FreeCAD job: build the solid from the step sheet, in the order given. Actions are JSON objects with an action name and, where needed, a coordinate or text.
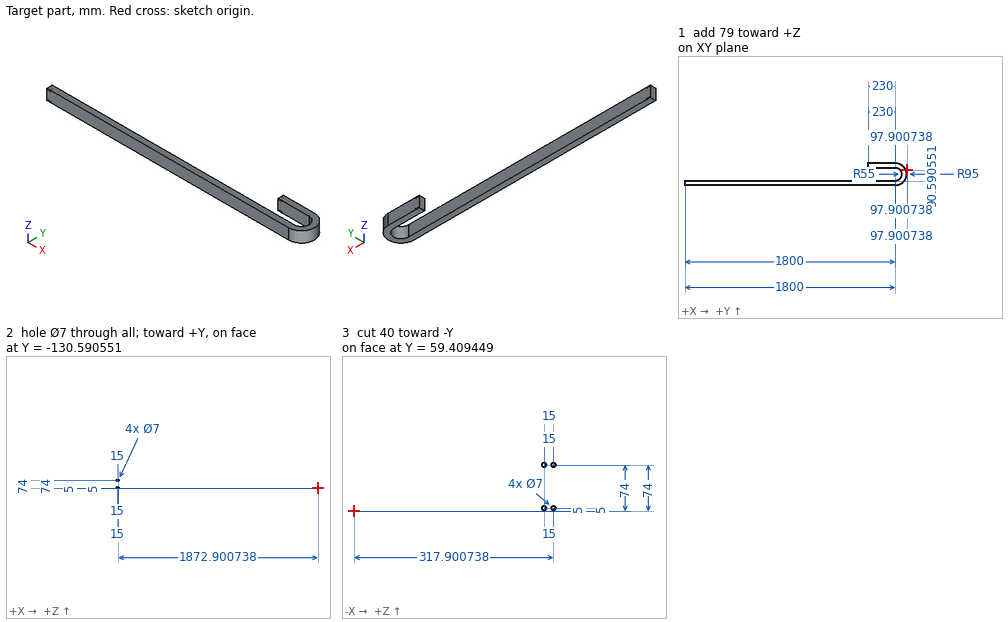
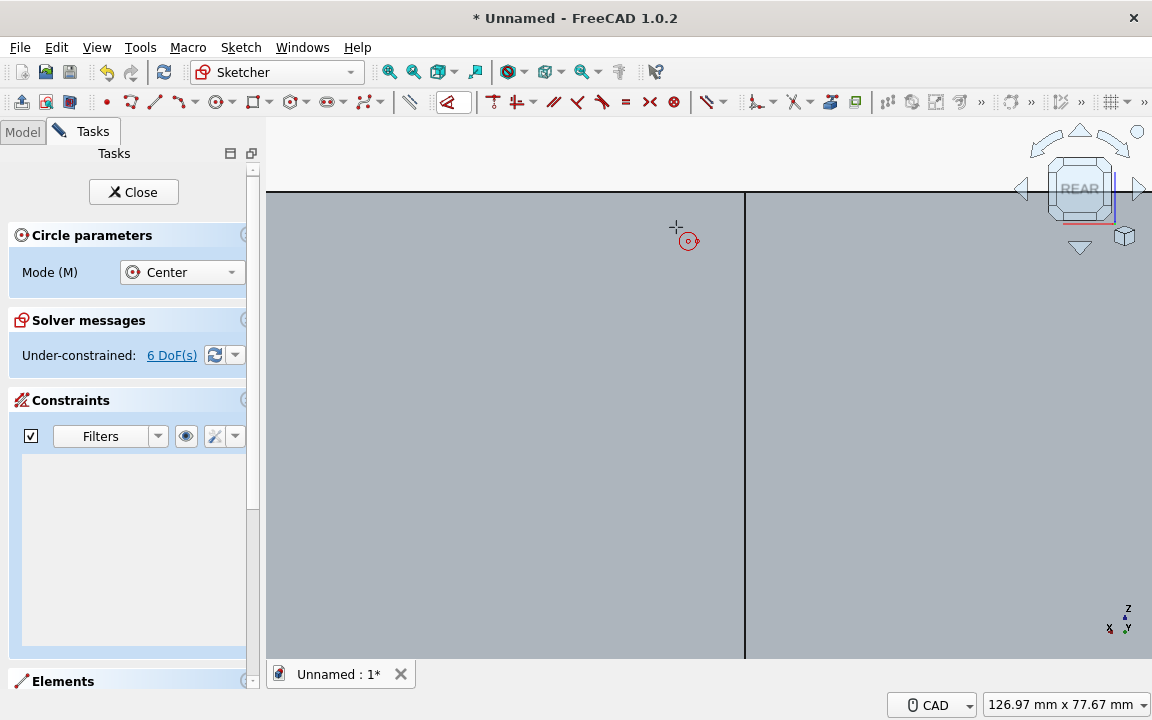
{"action": "left_click", "coordinate": [676, 227]}
{"action": "left_click", "coordinate": [693, 209]}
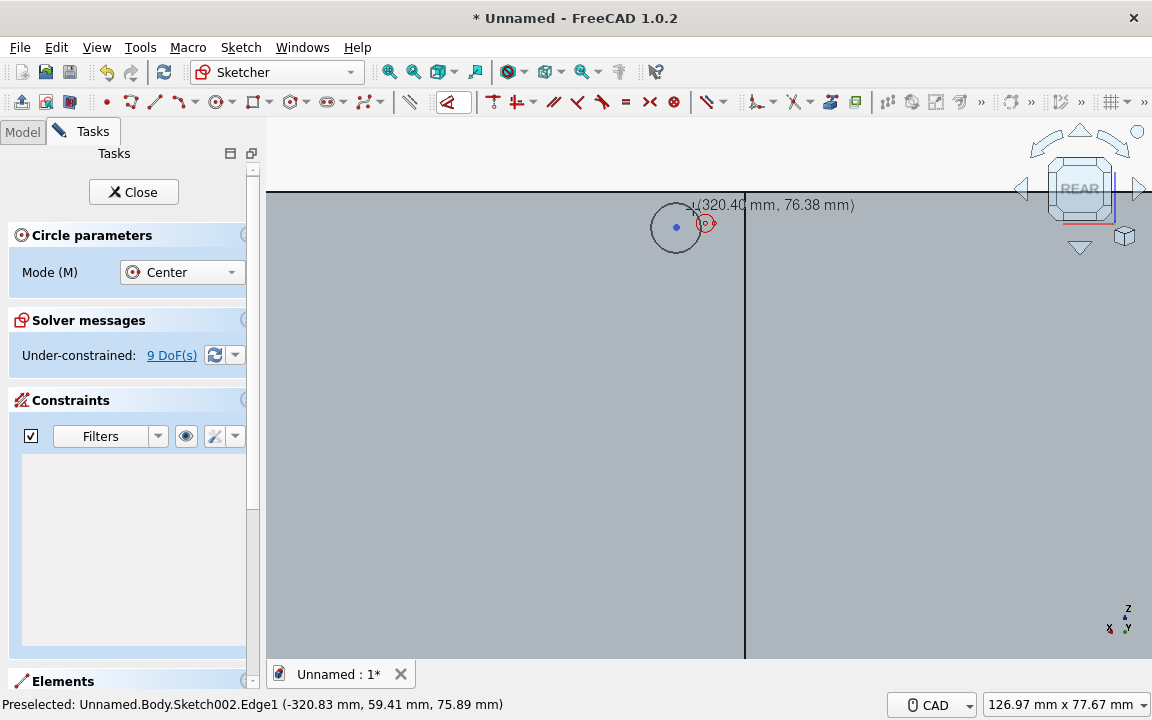
{"action": "left_click", "coordinate": [571, 227]}
{"action": "left_click", "coordinate": [588, 209]}
{"action": "key", "text": "Escape"}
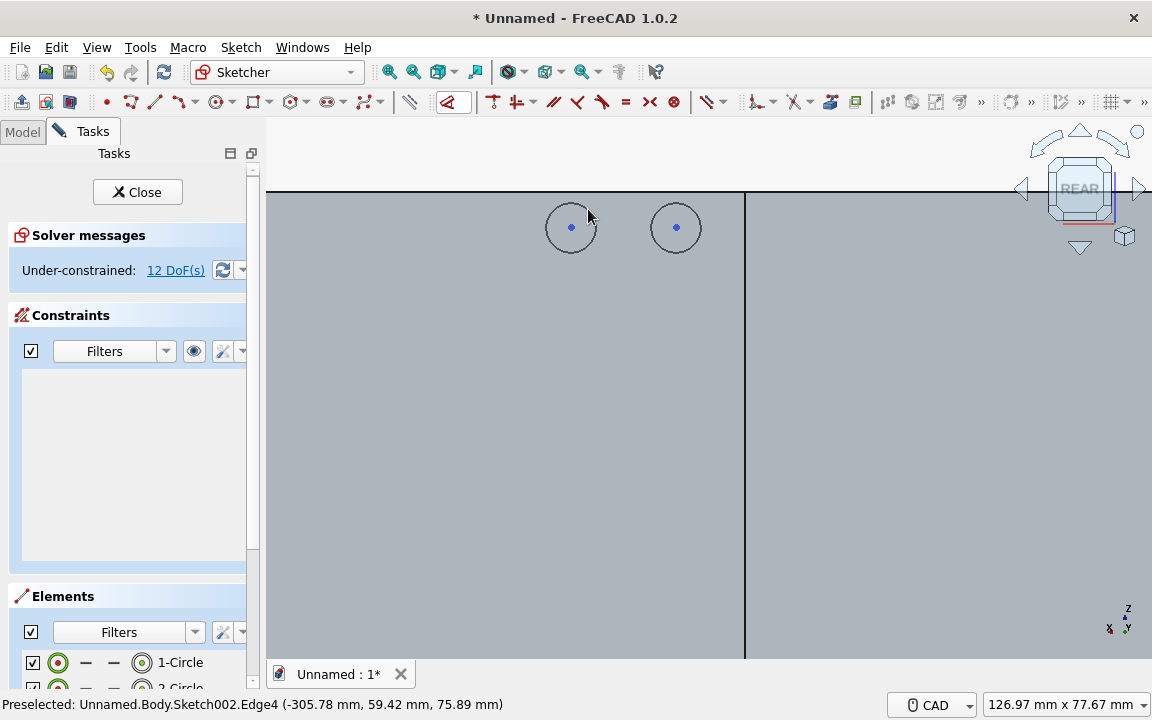
{"action": "scroll", "coordinate": [676, 227], "scroll_direction": "down", "scroll_amount": 2}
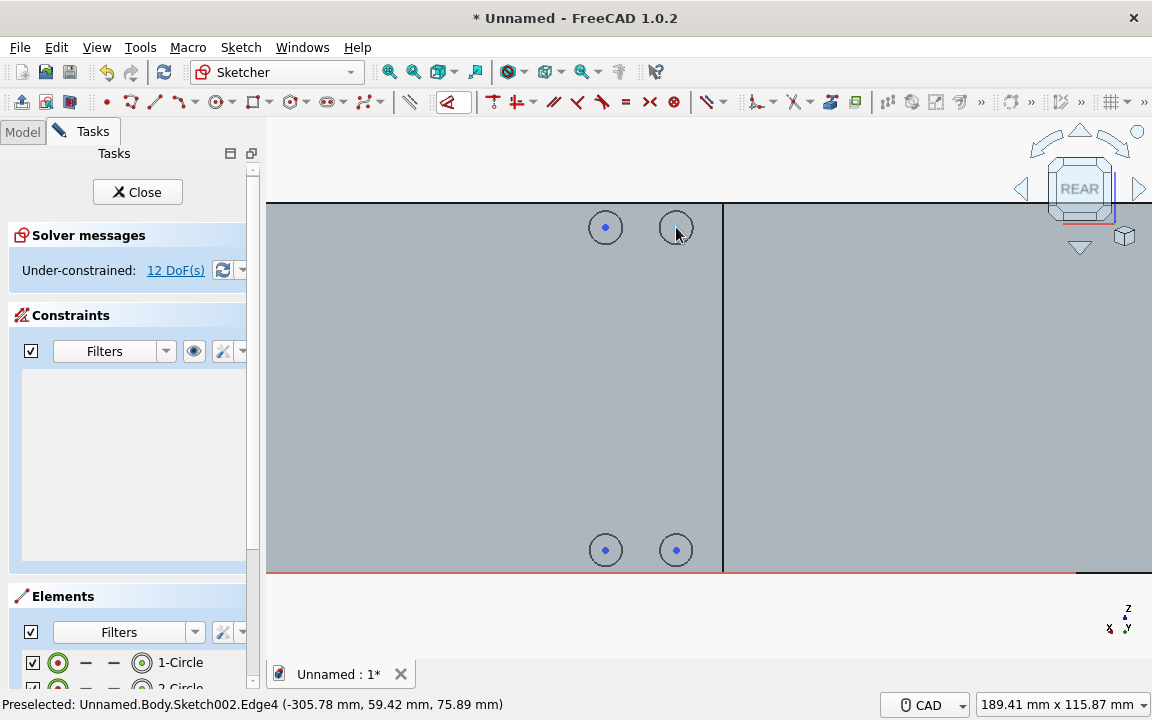
{"action": "left_click", "coordinate": [688, 539]}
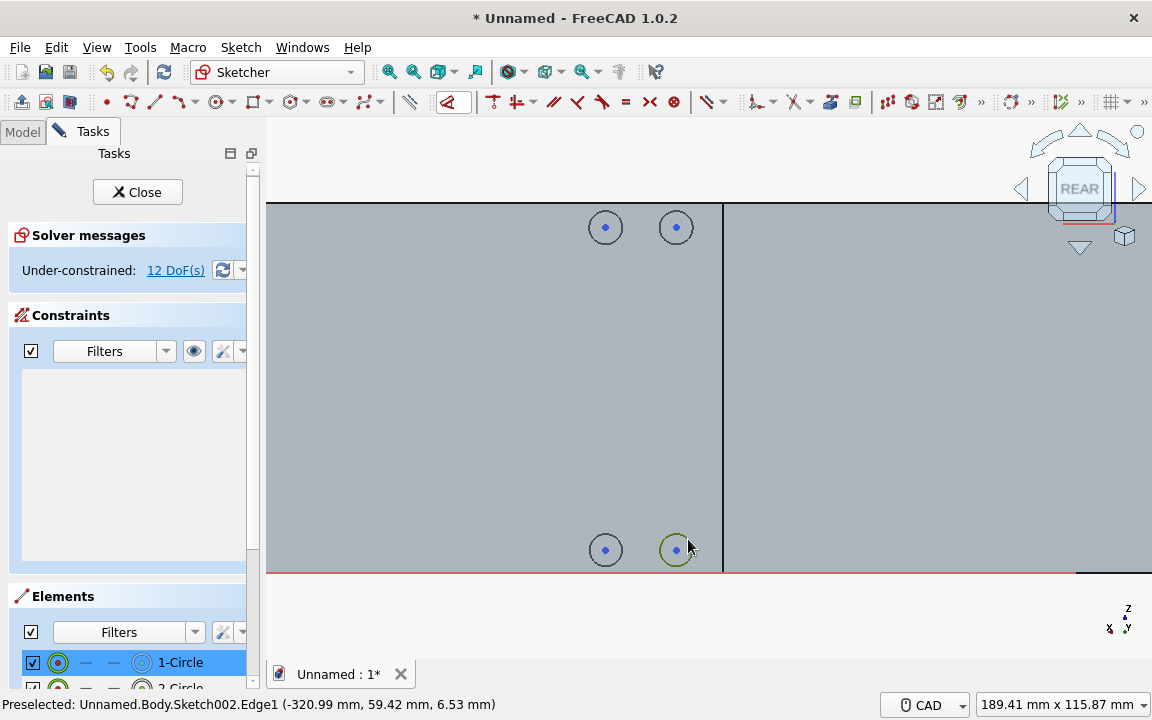
{"action": "left_click", "coordinate": [617, 539]}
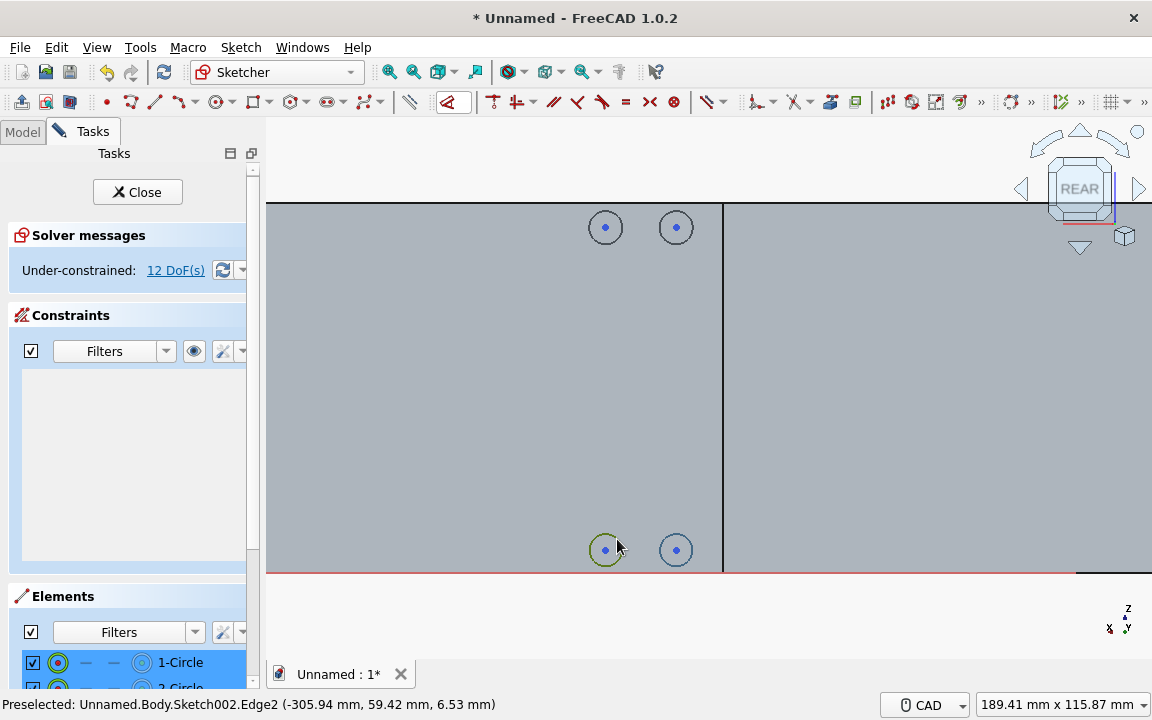
{"action": "left_click", "coordinate": [688, 216]}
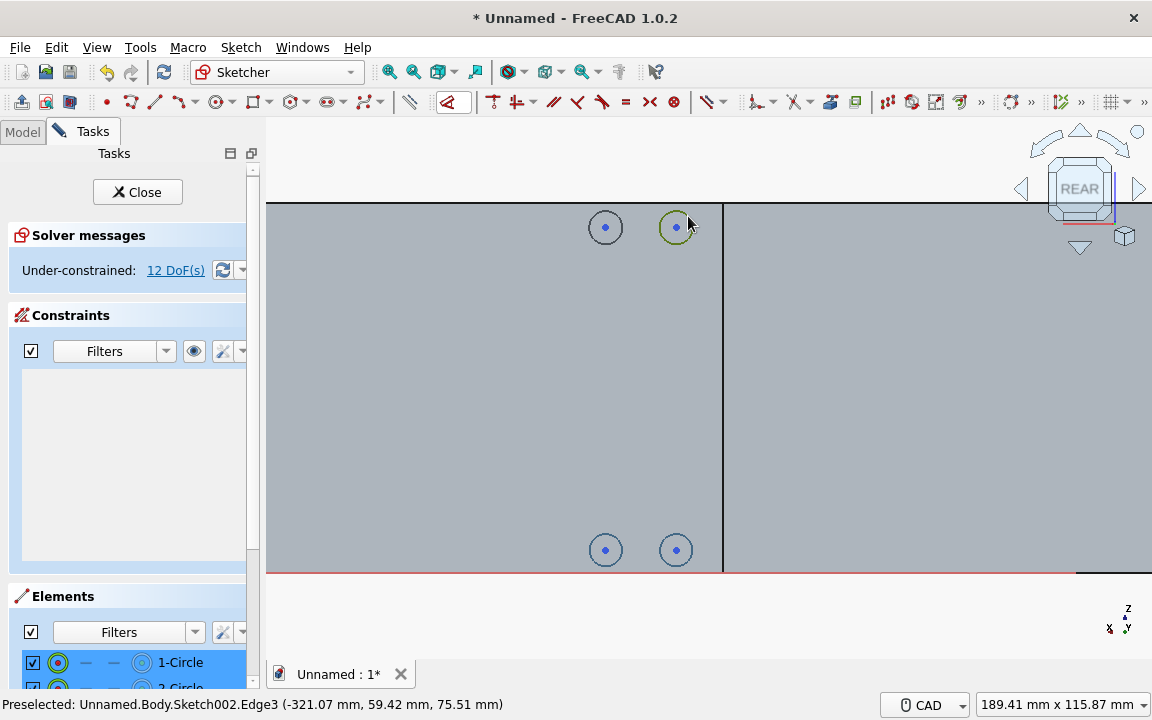
{"action": "left_click", "coordinate": [617, 216]}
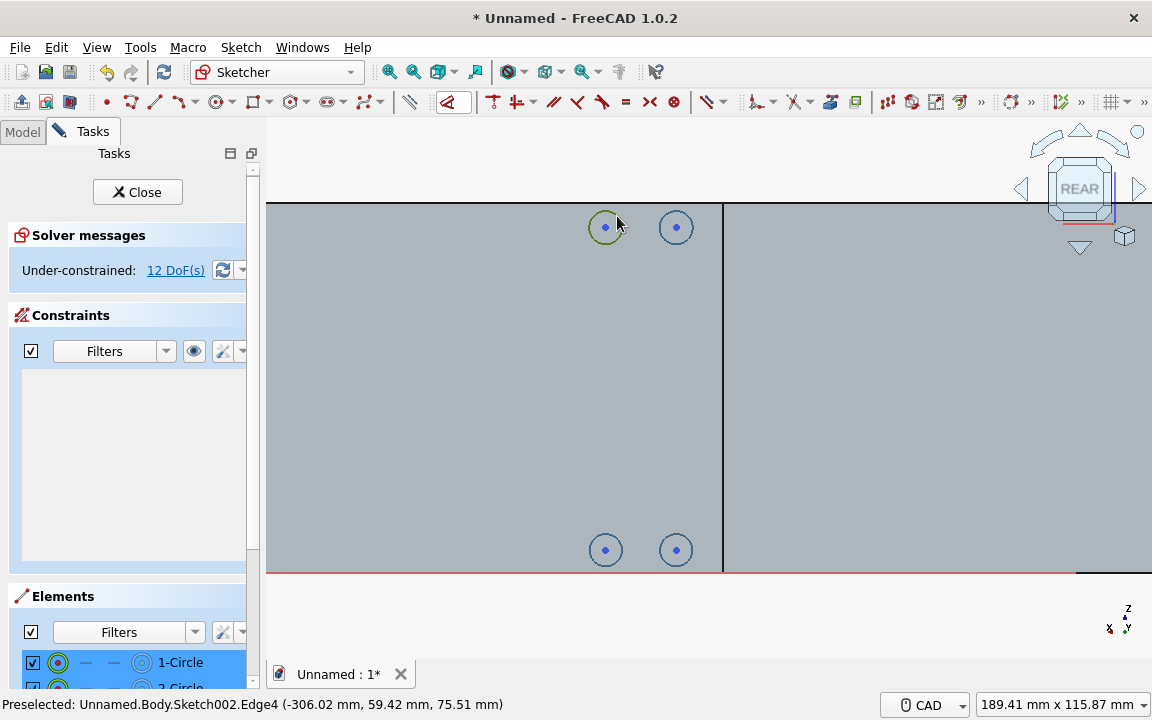
{"action": "key", "text": "e"}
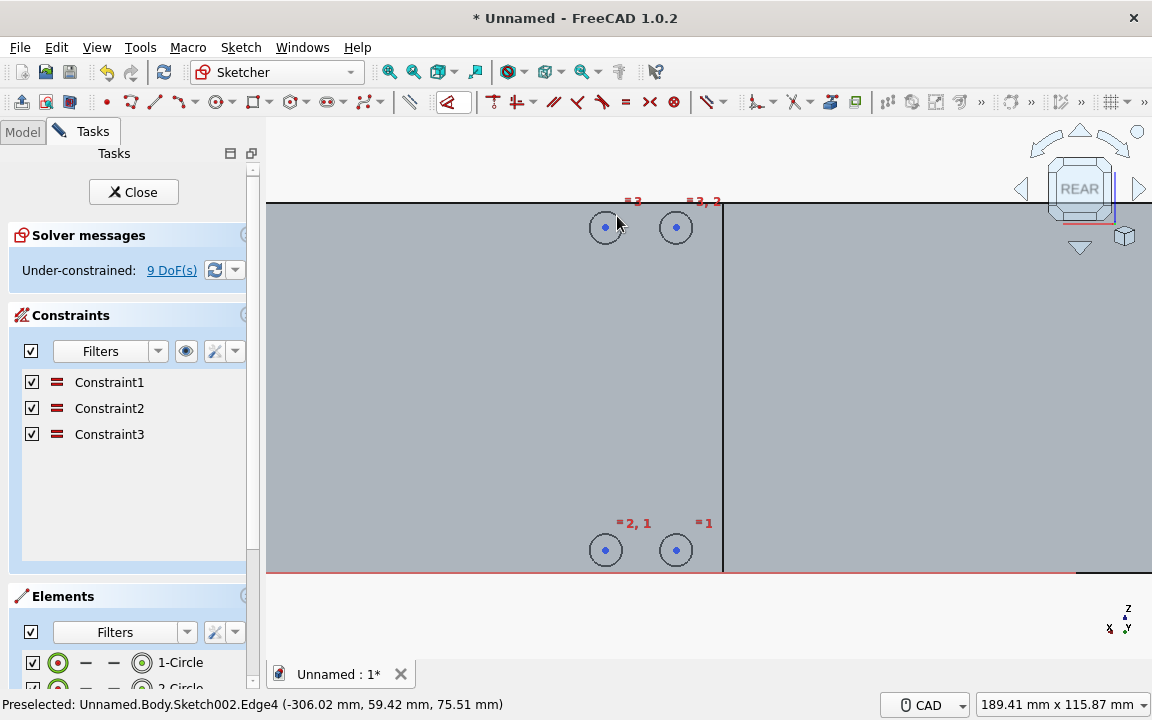
{"action": "key", "text": "d"}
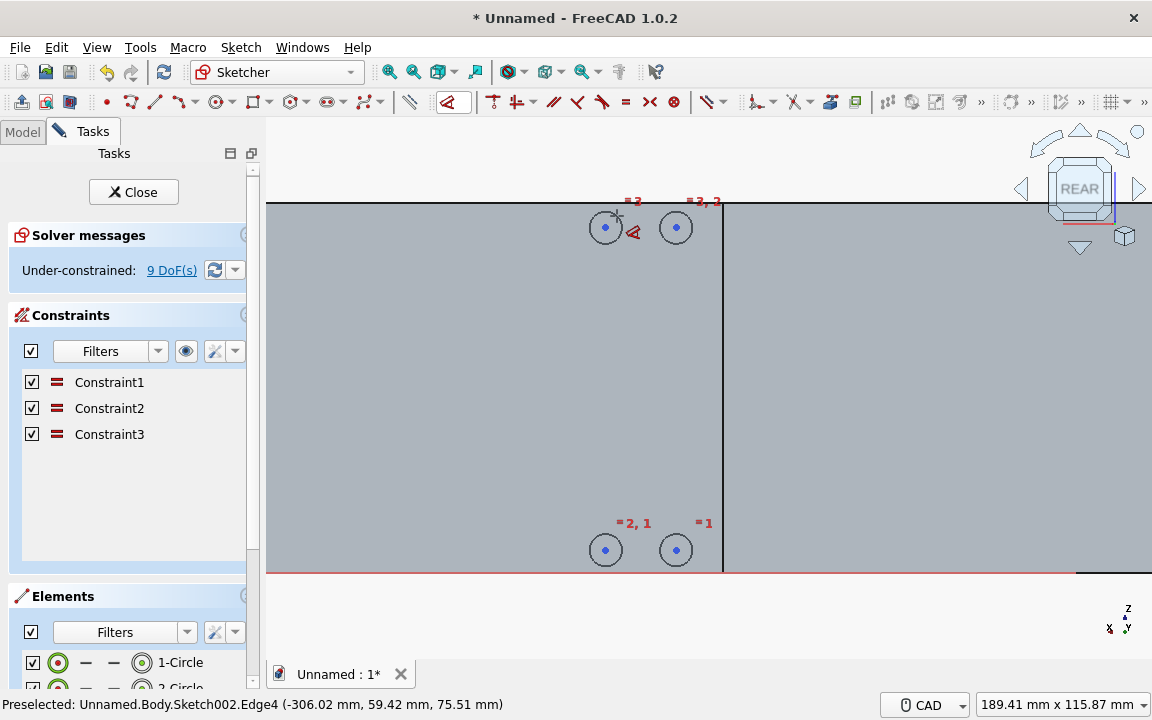
{"action": "left_click", "coordinate": [688, 539]}
{"action": "left_click", "coordinate": [711, 517]}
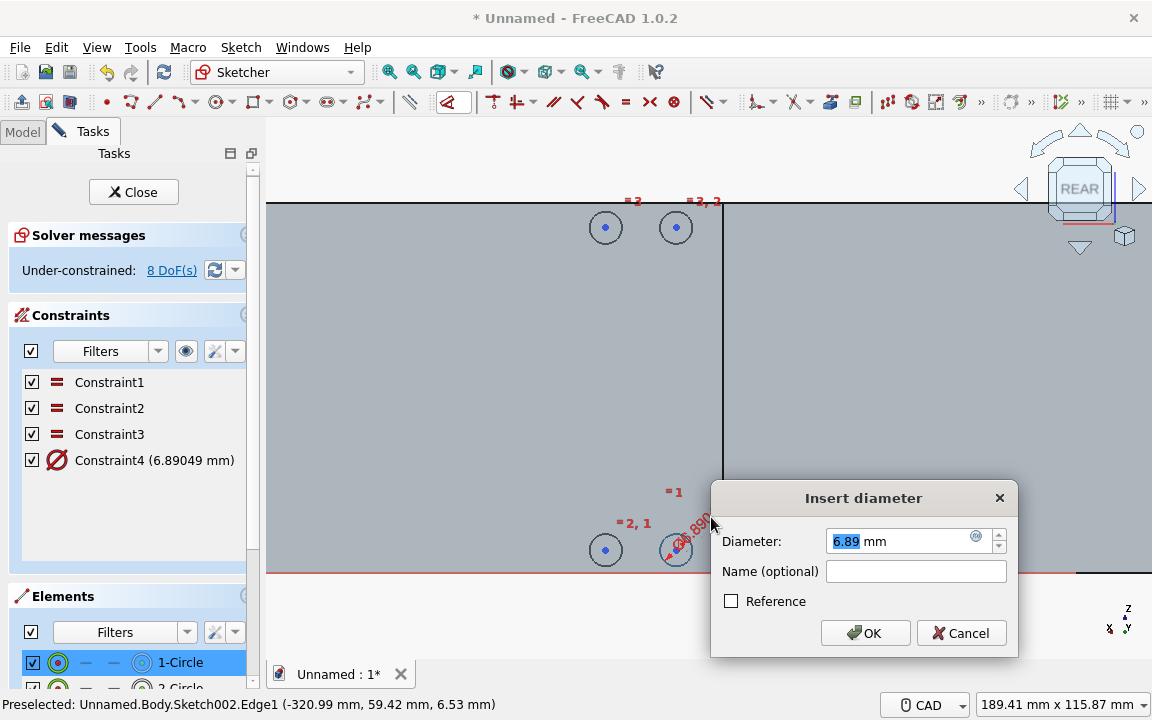
{"action": "type", "text": "7"}
{"action": "key", "text": "Return"}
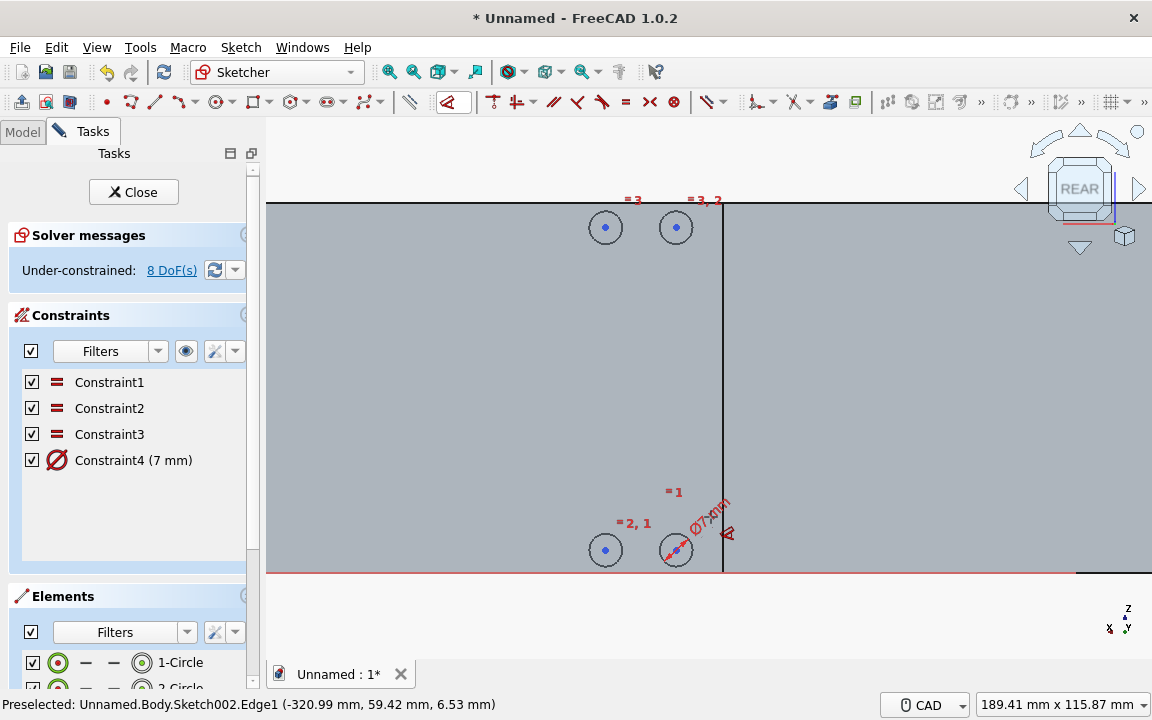
{"action": "scroll", "coordinate": [676, 550], "scroll_direction": "up", "scroll_amount": 3}